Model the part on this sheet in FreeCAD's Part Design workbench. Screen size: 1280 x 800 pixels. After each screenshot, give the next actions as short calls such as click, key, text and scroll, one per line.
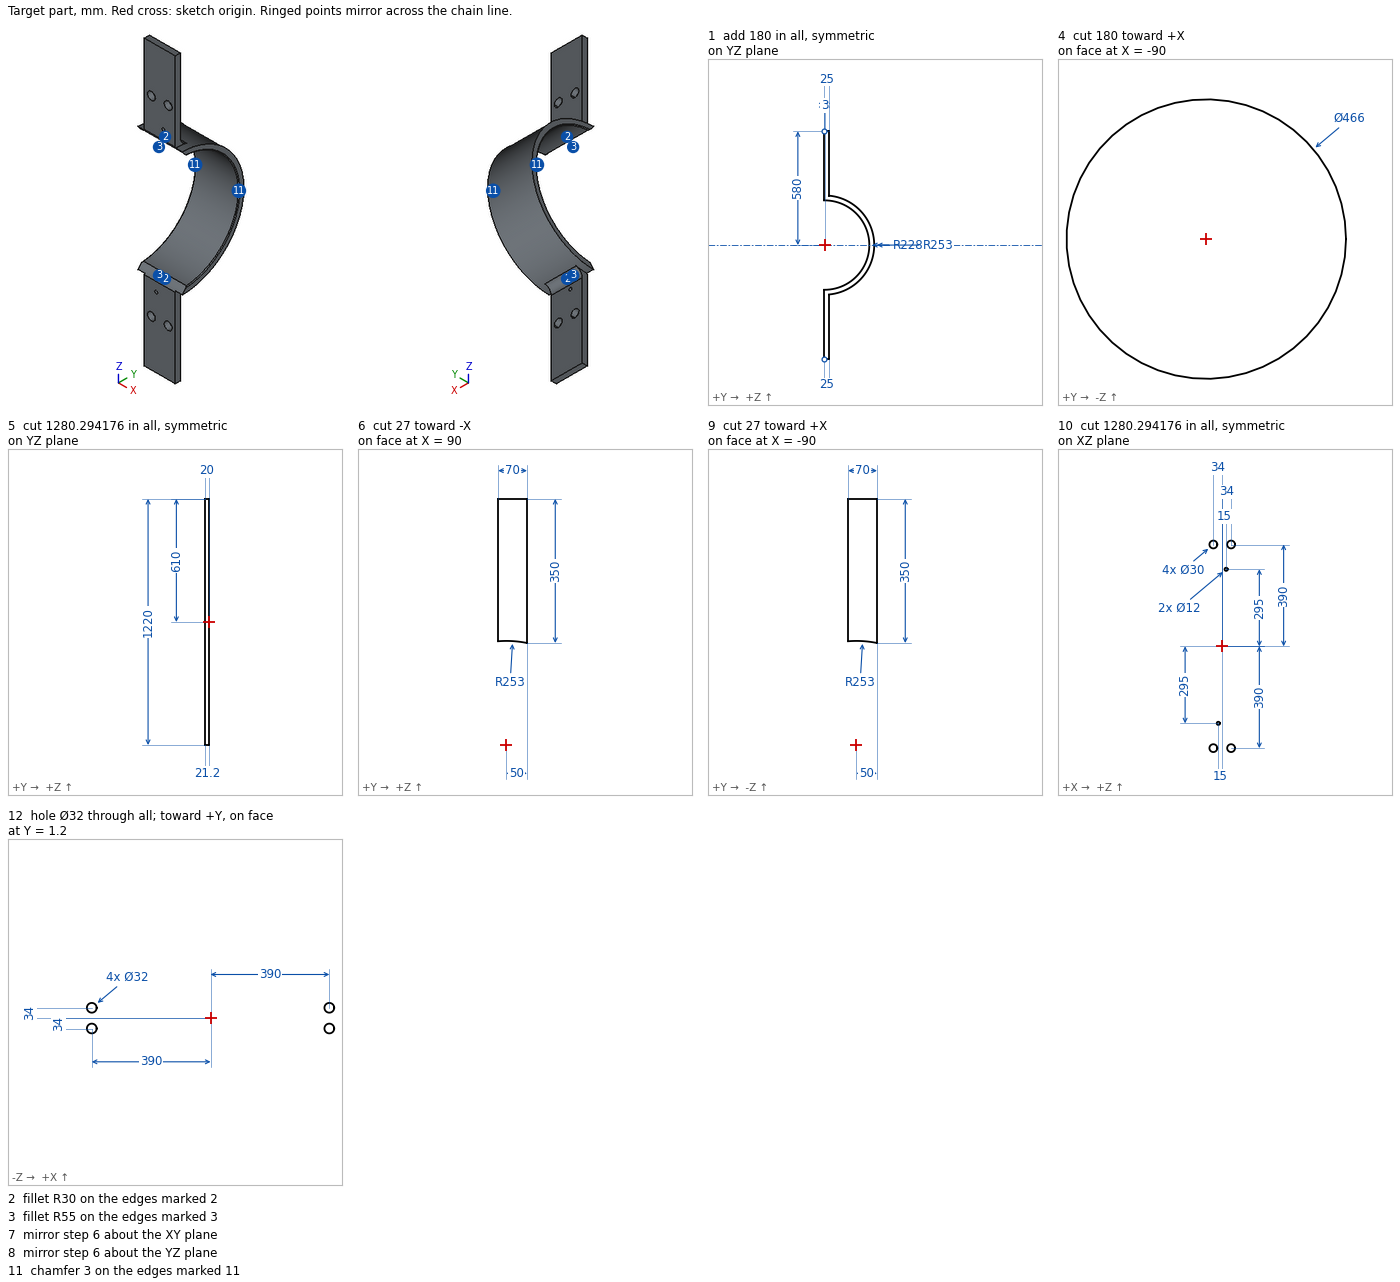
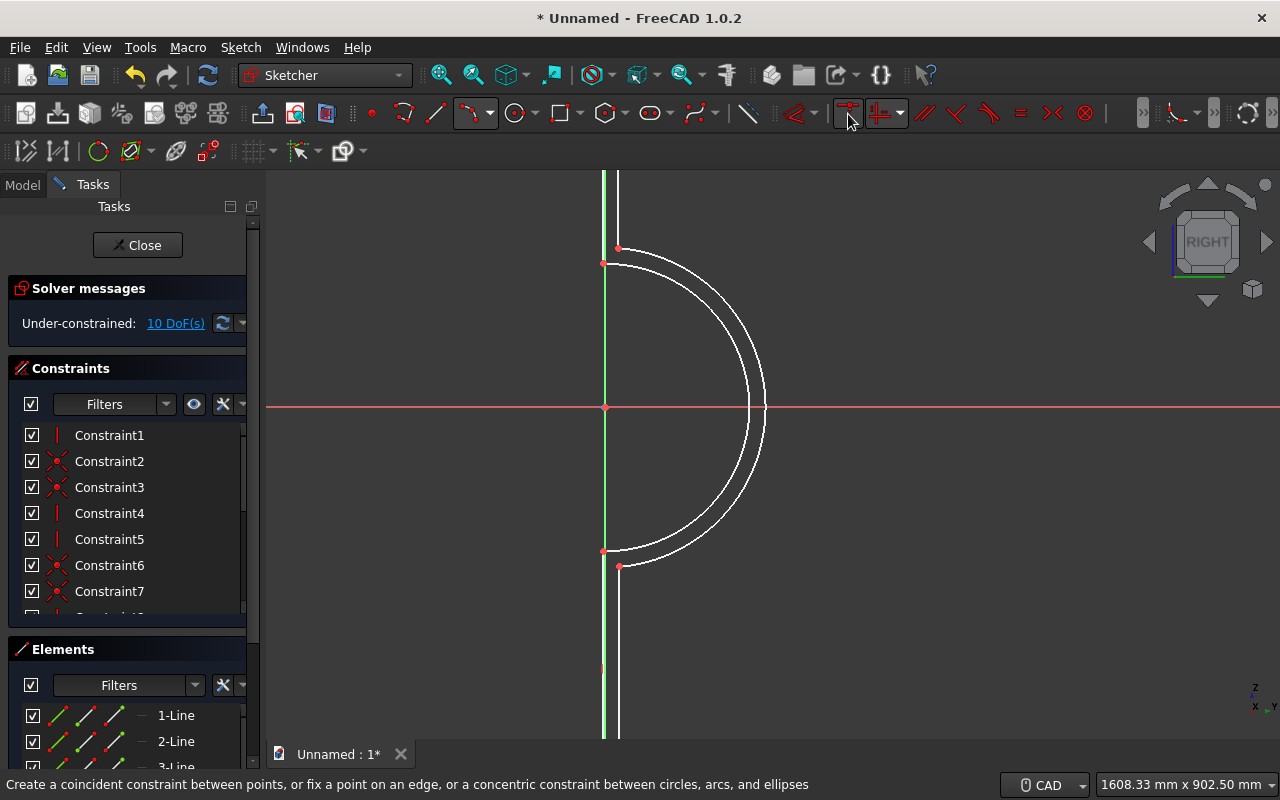
drag(595, 397, 616, 418)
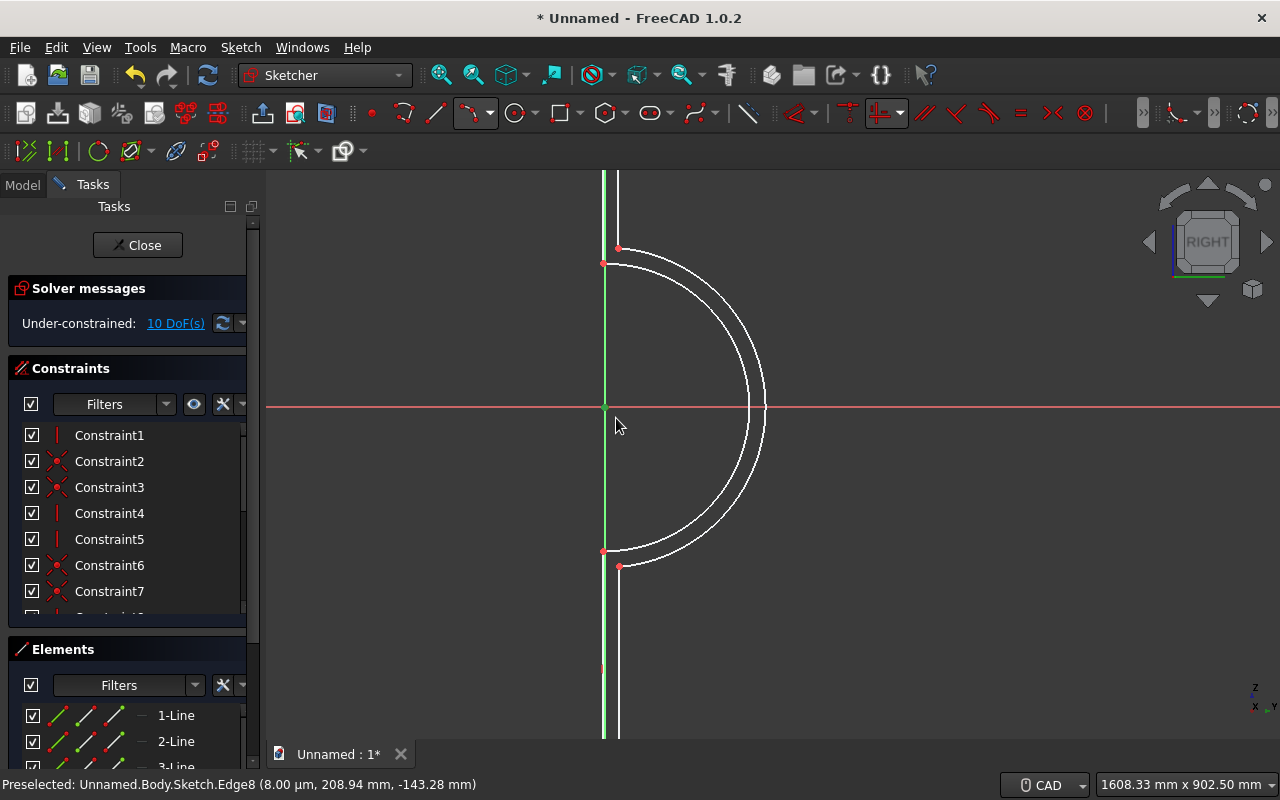
click(848, 114)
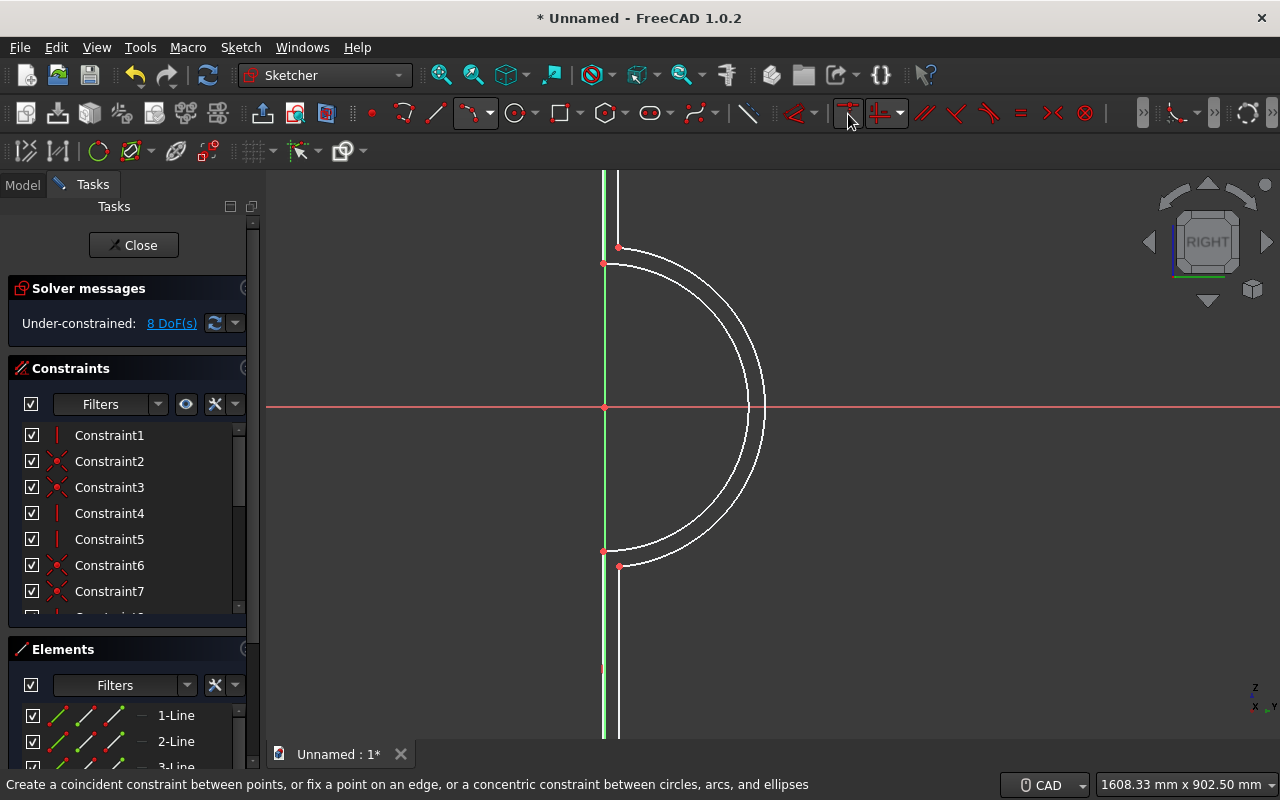
scroll(721, 493, down, 4)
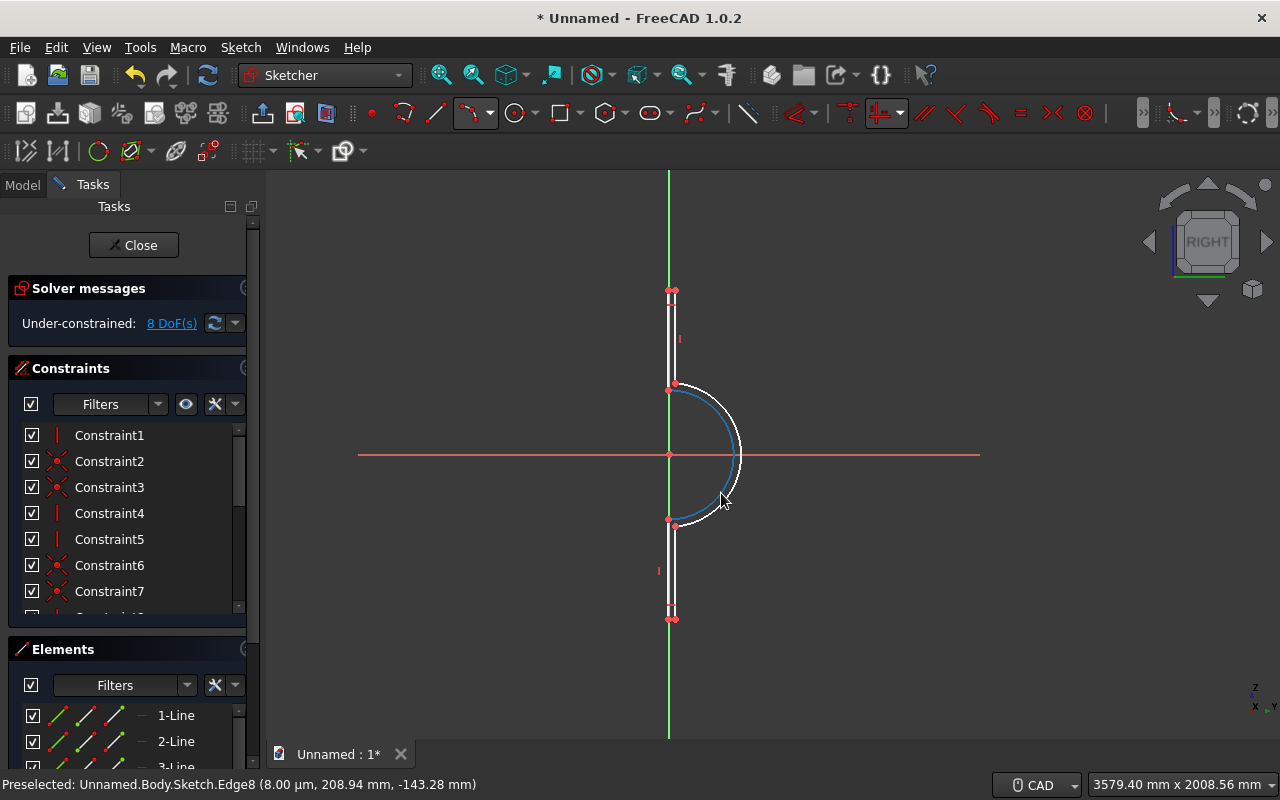
scroll(668, 291, up, 3)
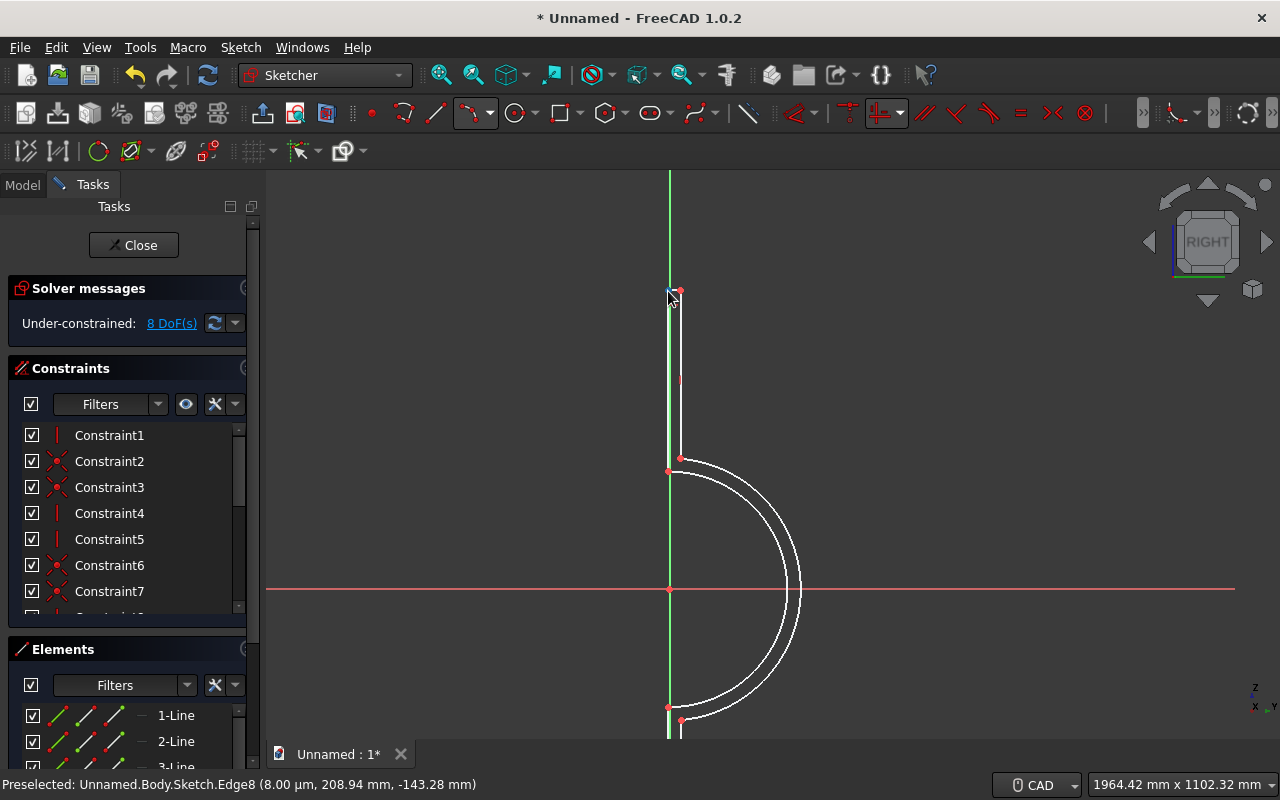
click(668, 290)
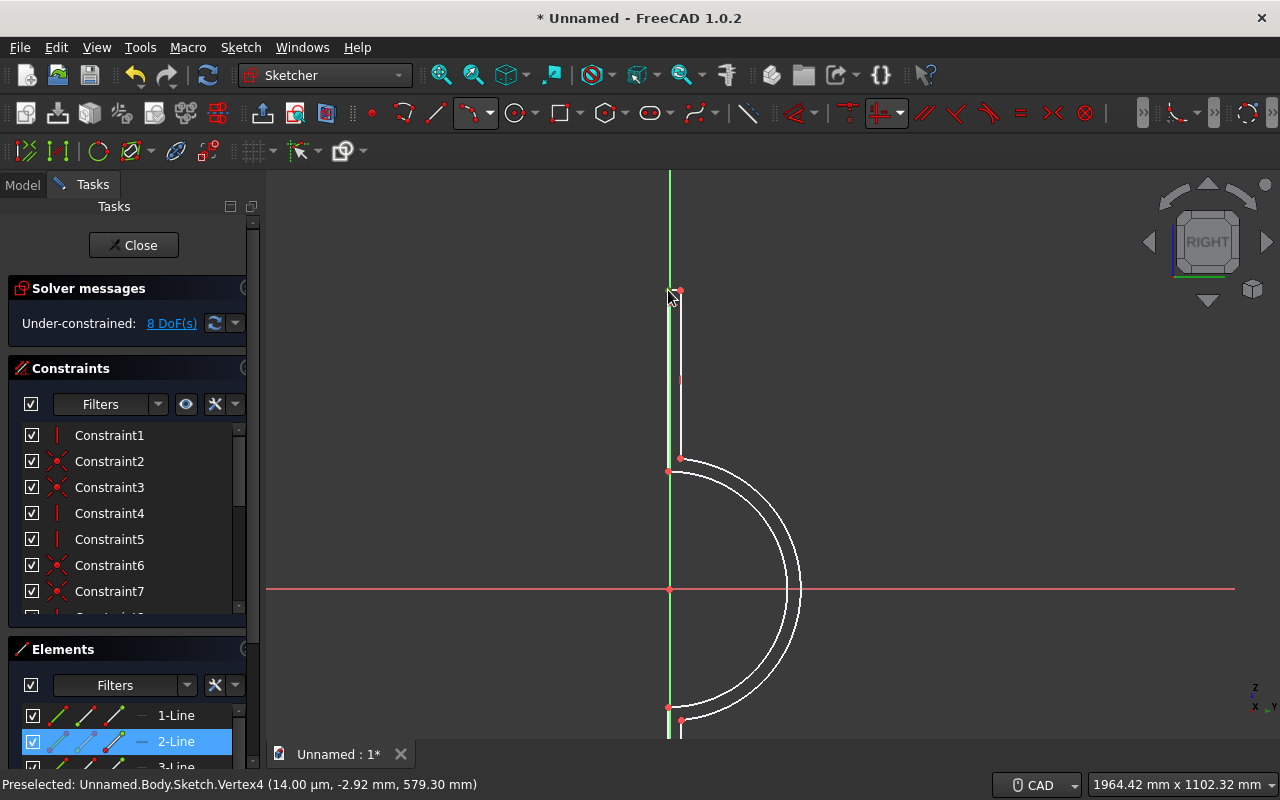
scroll(668, 290, down, 3)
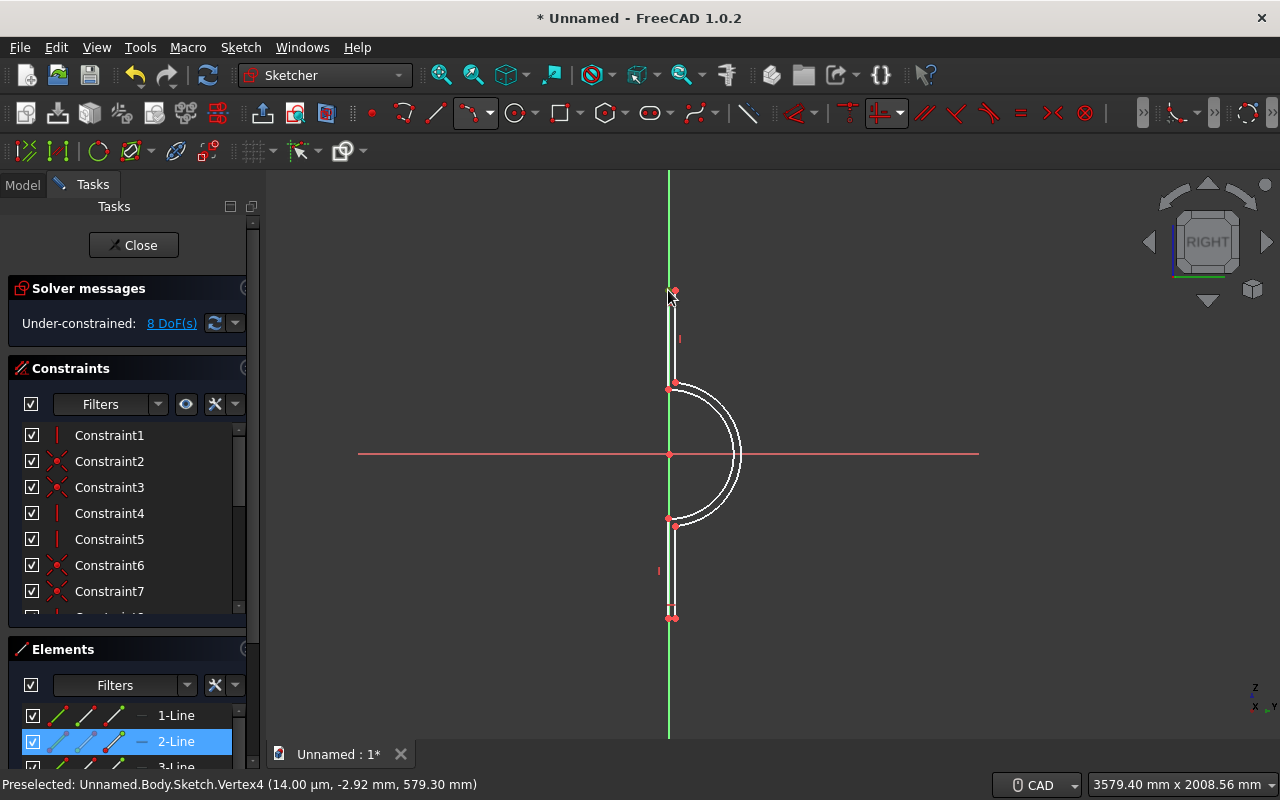
scroll(668, 619, up, 3)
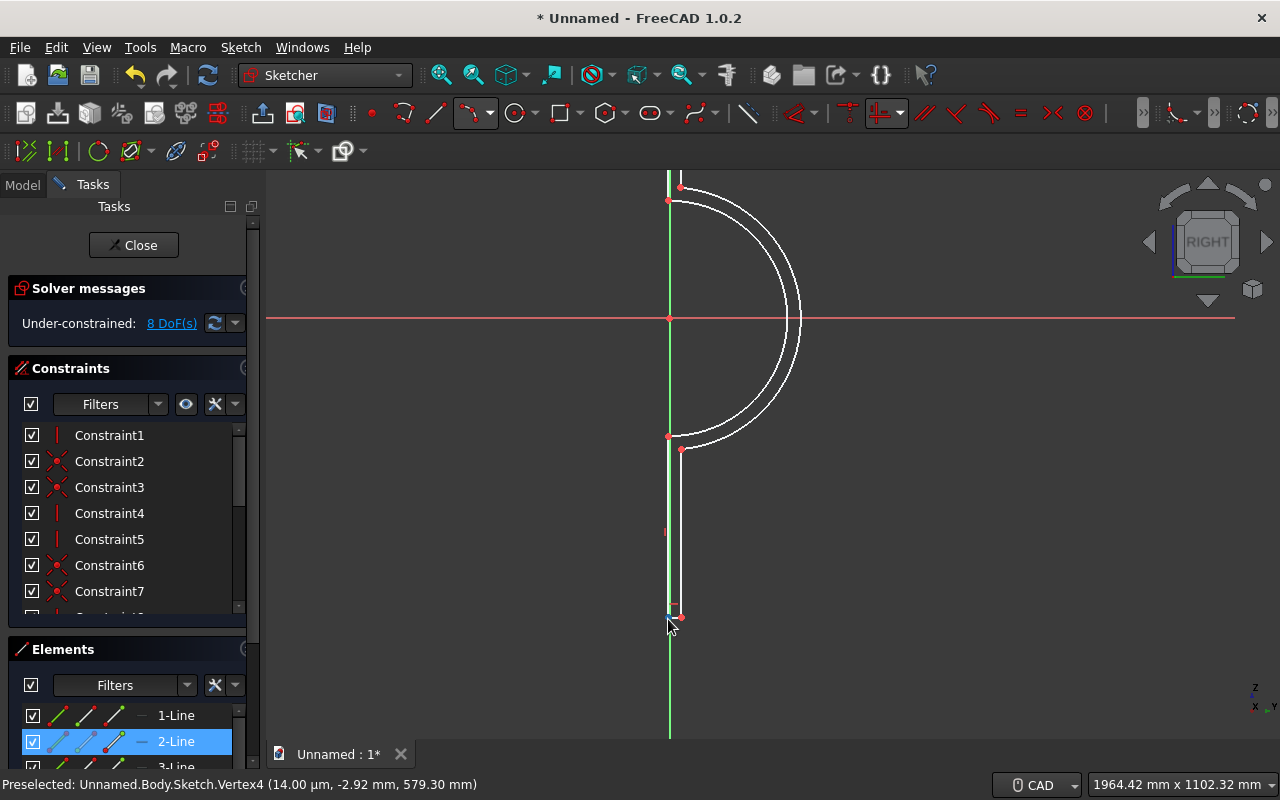
click(668, 618)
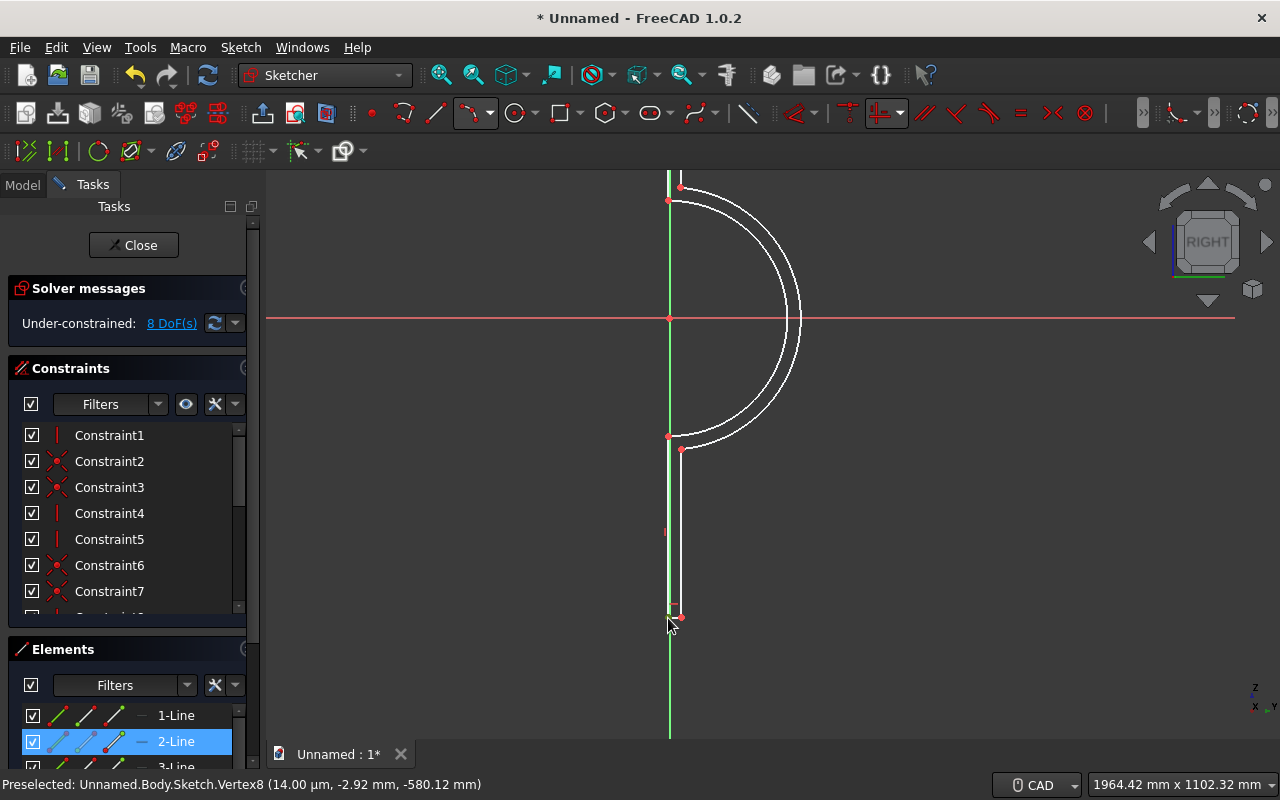
click(353, 318)